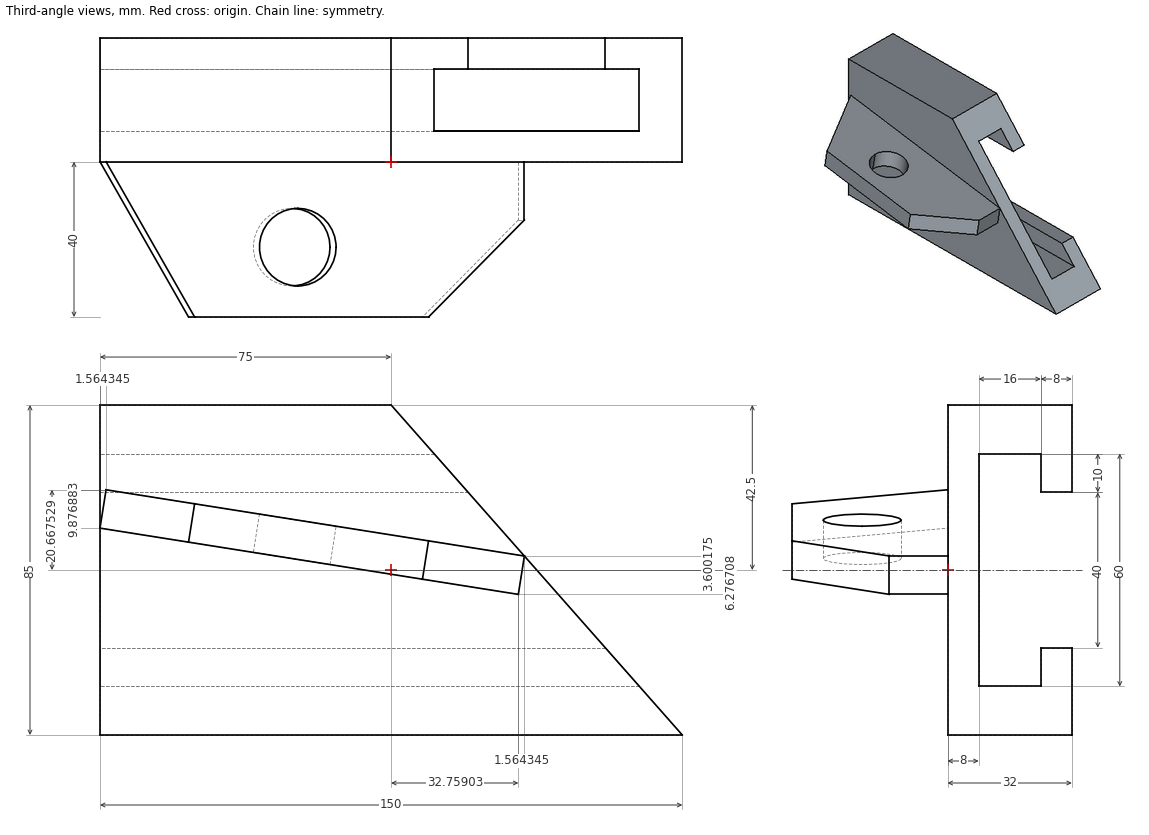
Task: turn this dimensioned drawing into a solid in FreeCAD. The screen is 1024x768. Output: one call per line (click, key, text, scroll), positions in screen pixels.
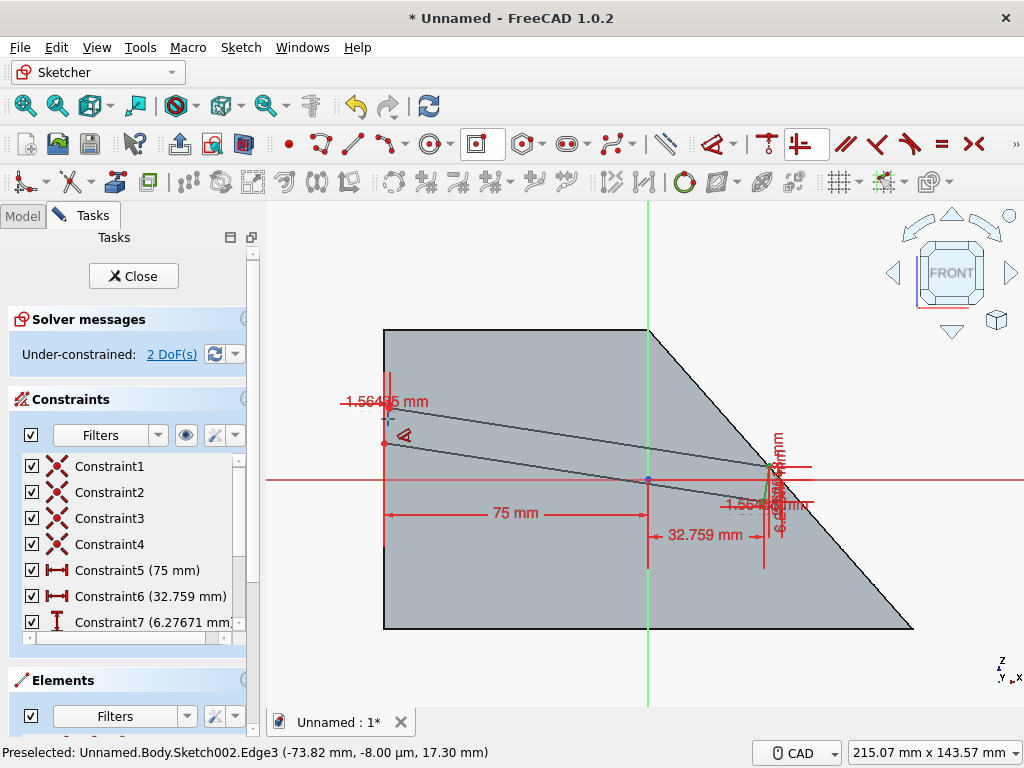
scroll(388, 419, up, 2)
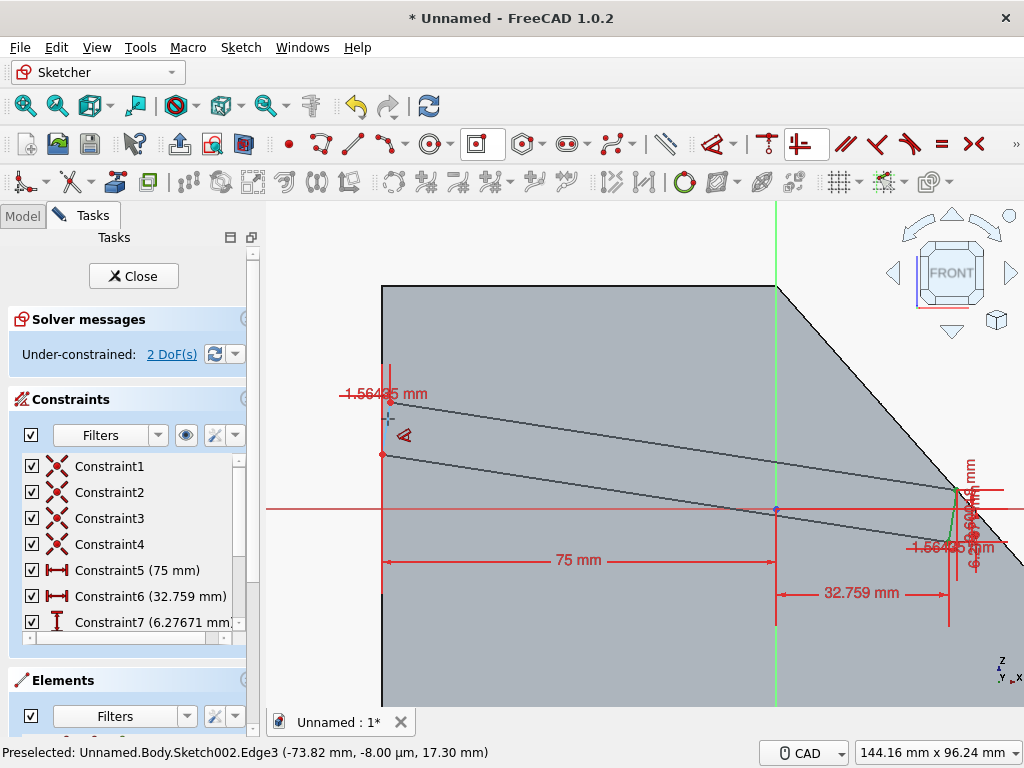
click(388, 418)
click(348, 429)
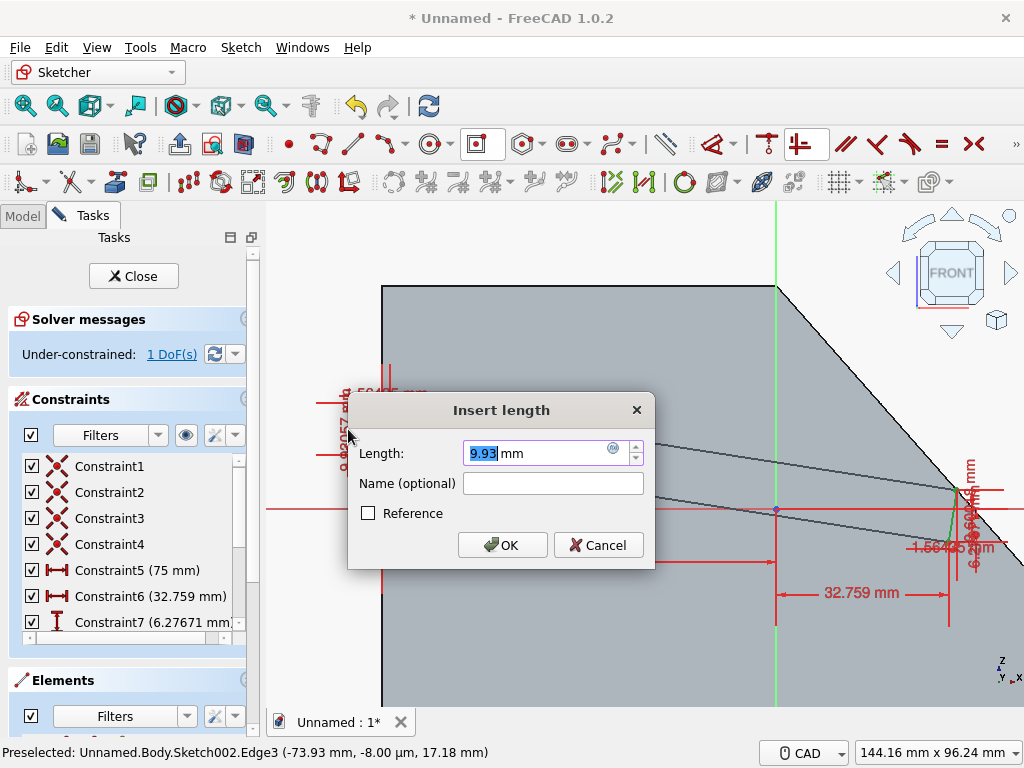
text(9.876883)
key(Return)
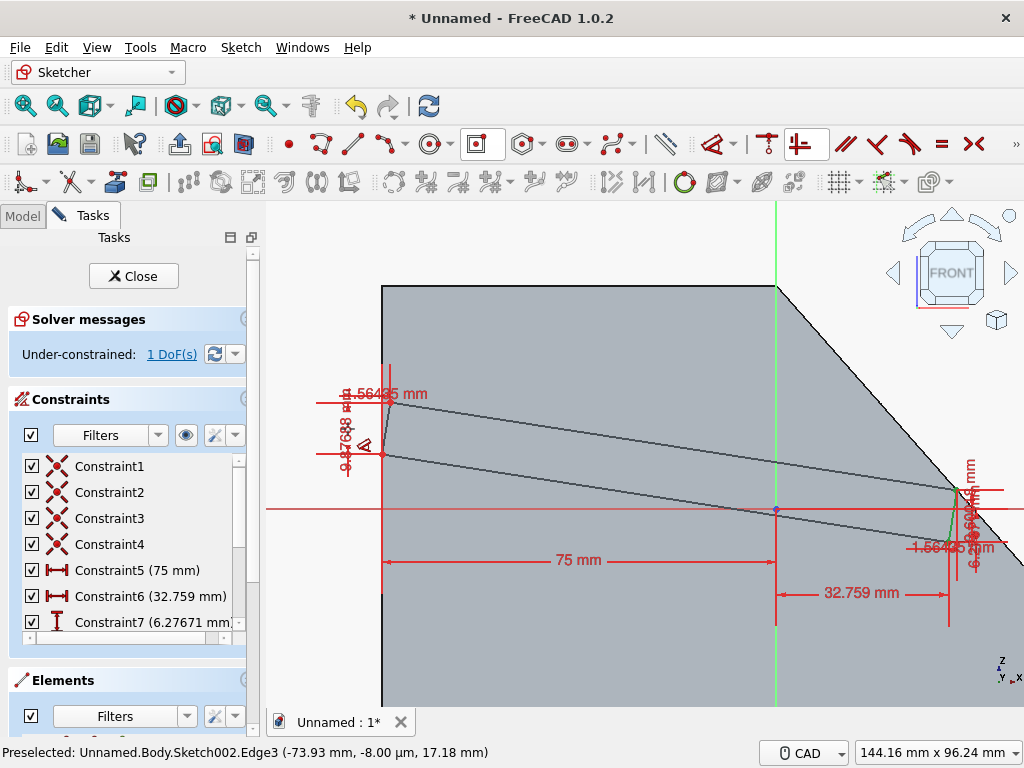
click(390, 403)
click(356, 456)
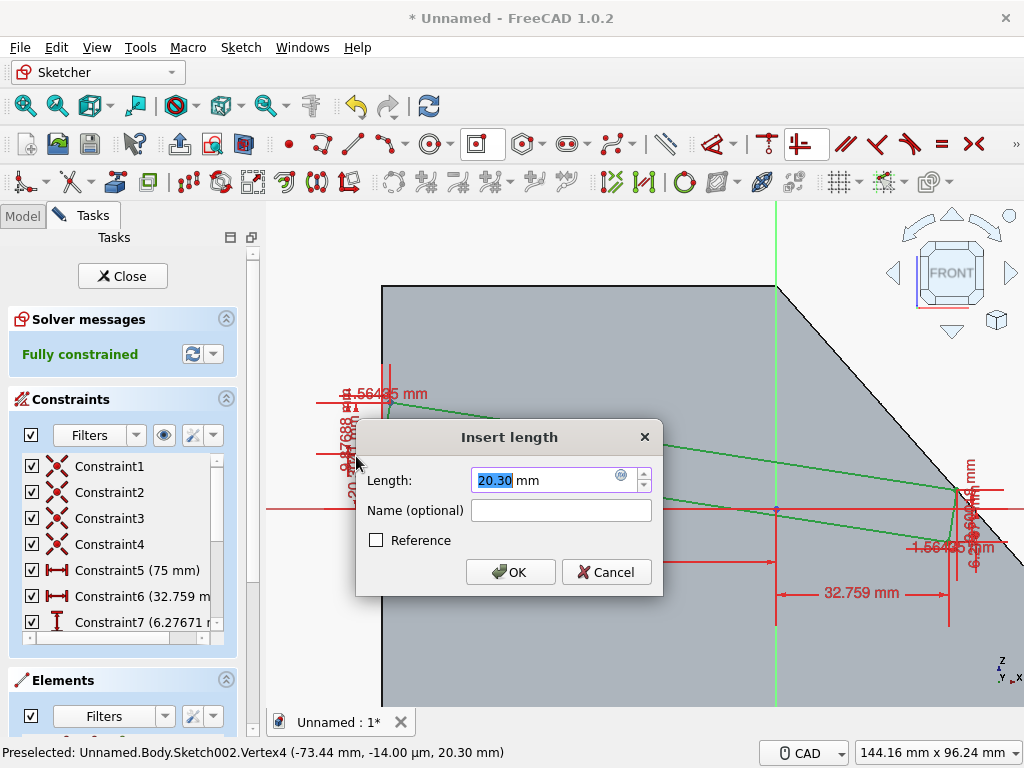
text(20.667529)
key(Return)
key(Escape)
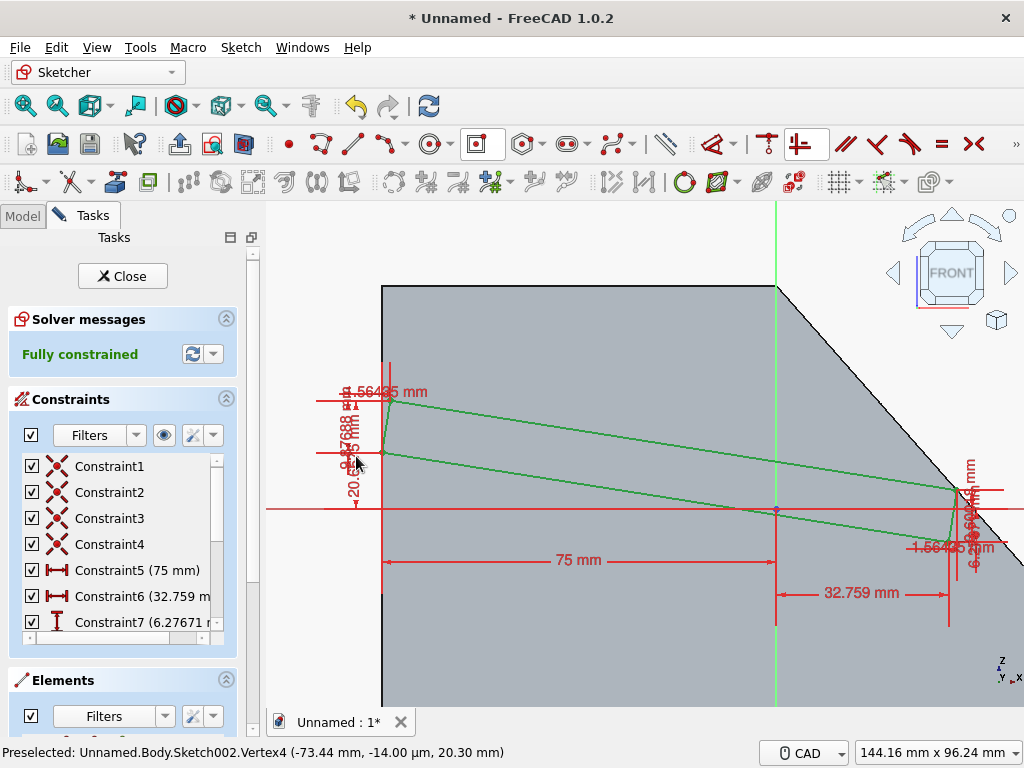
click(123, 276)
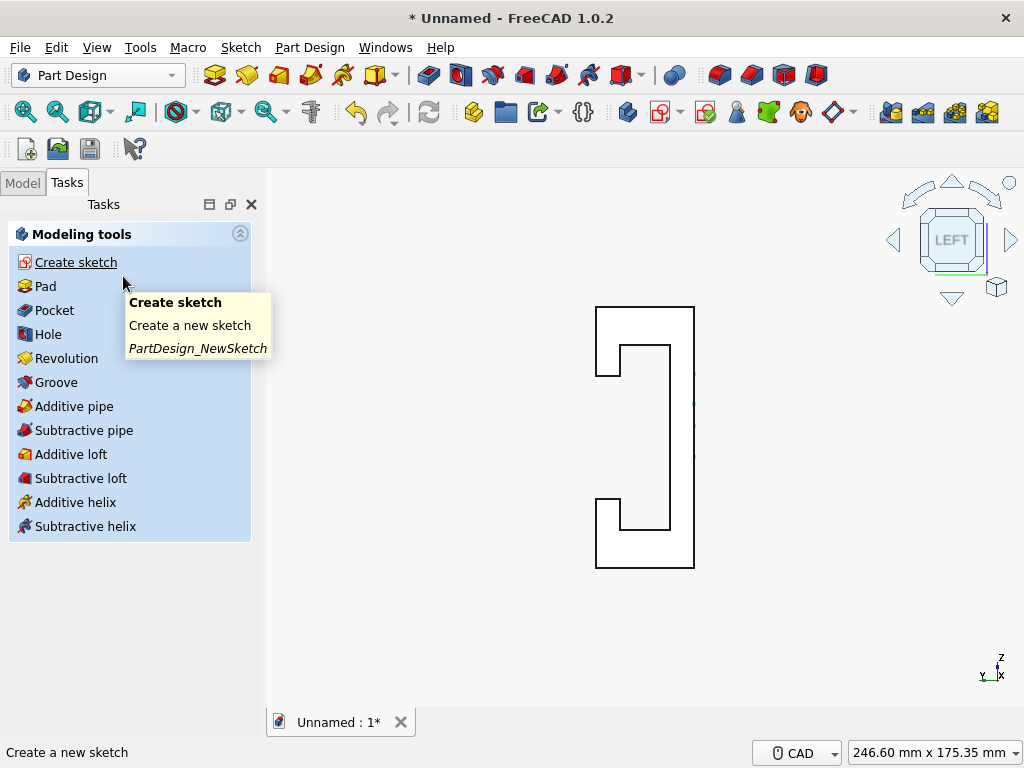
click(216, 76)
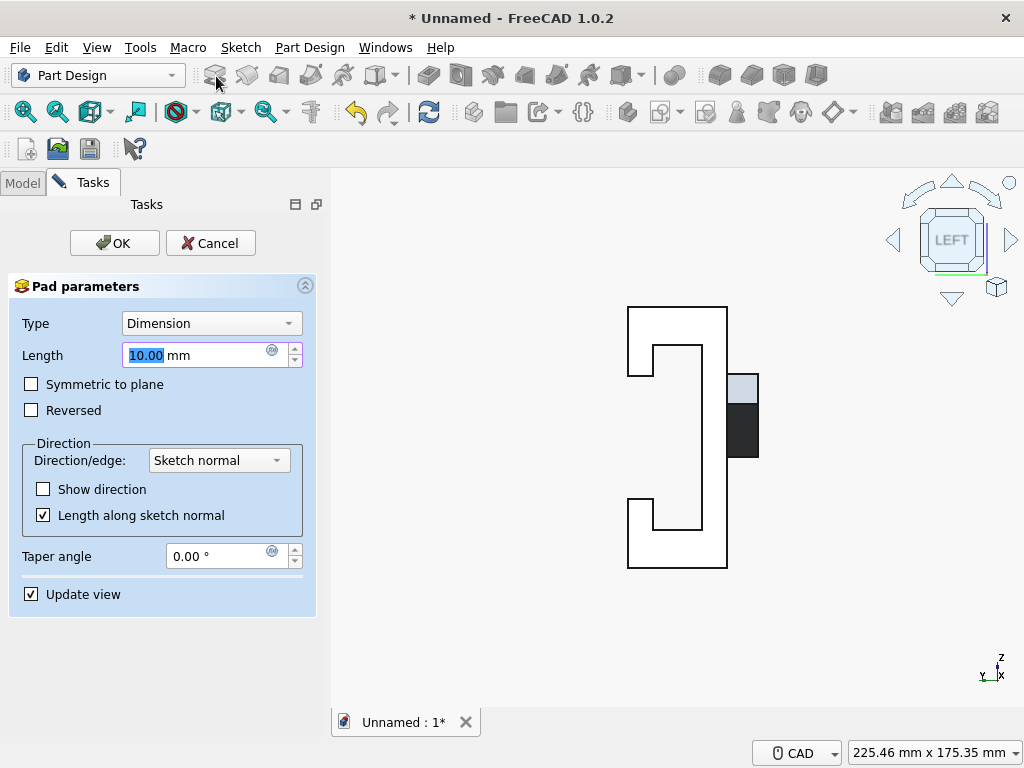
text(40)
key(Tab)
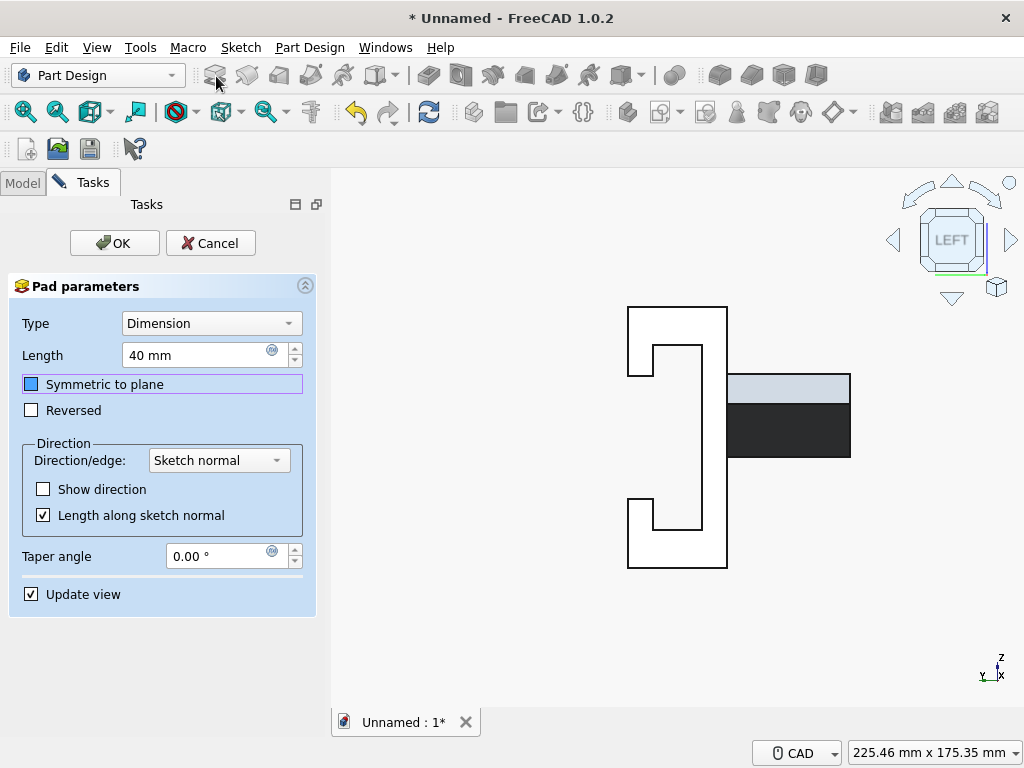
click(115, 243)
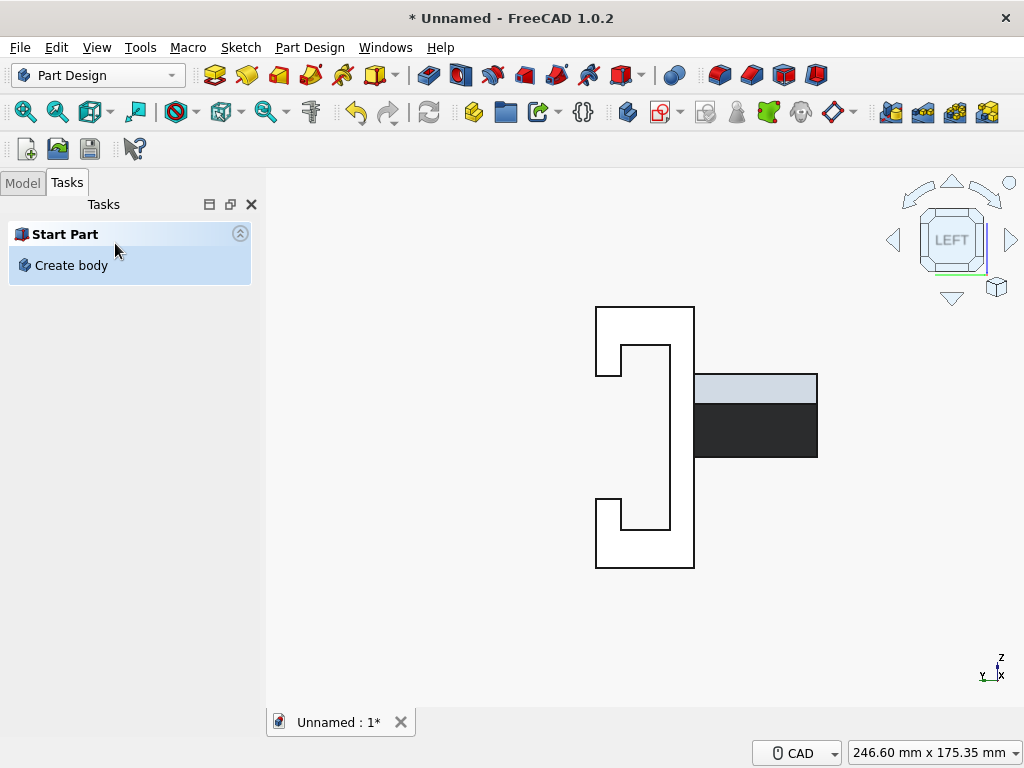
key(0)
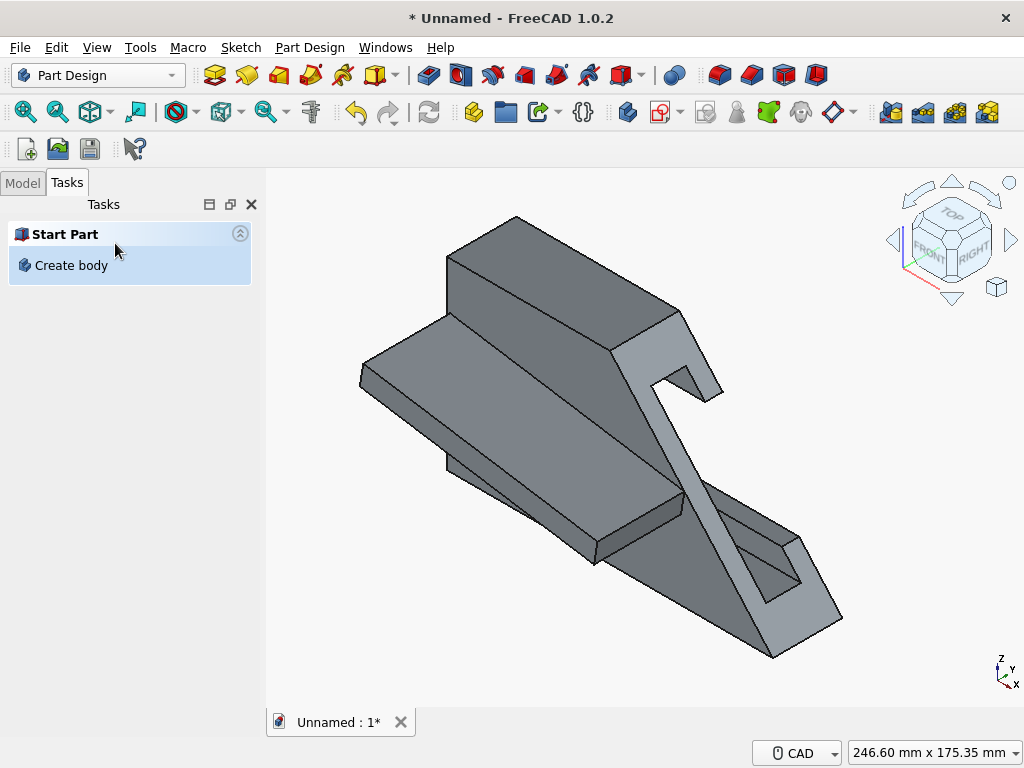
click(591, 477)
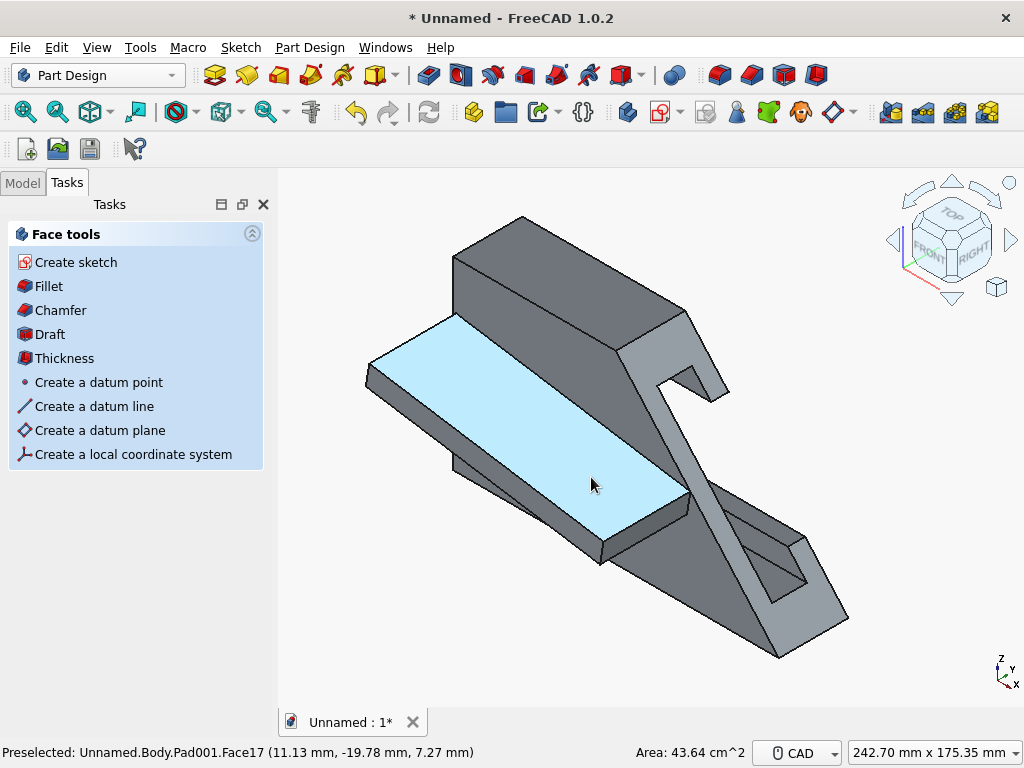
click(660, 112)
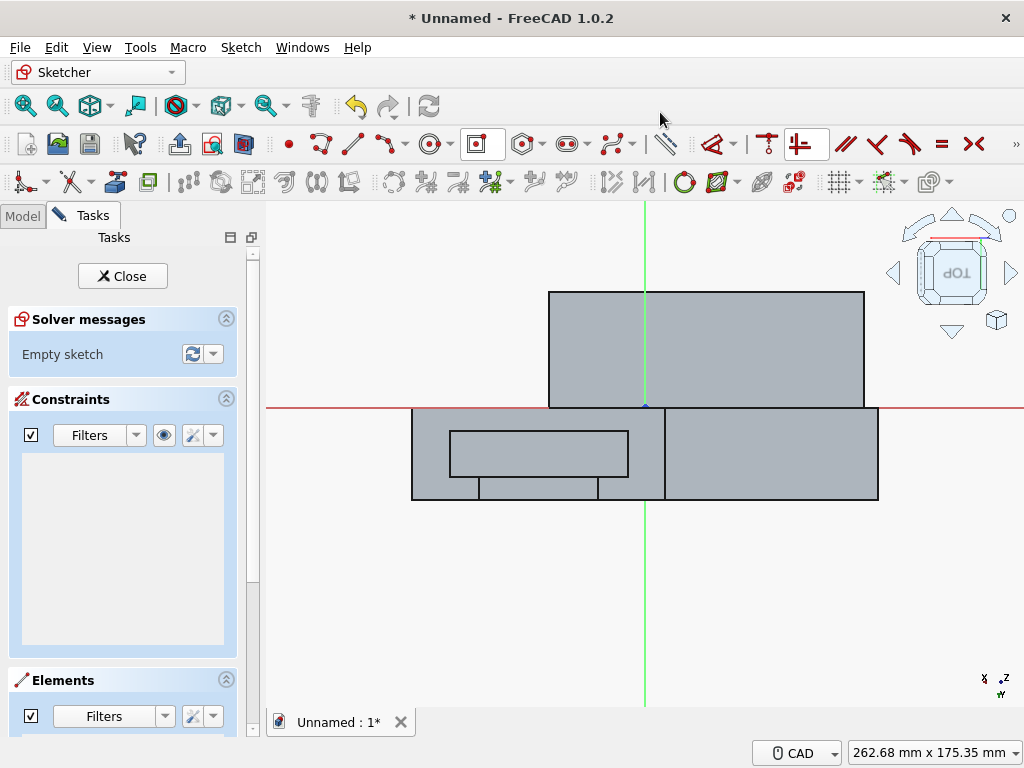
key(q)
key(s)